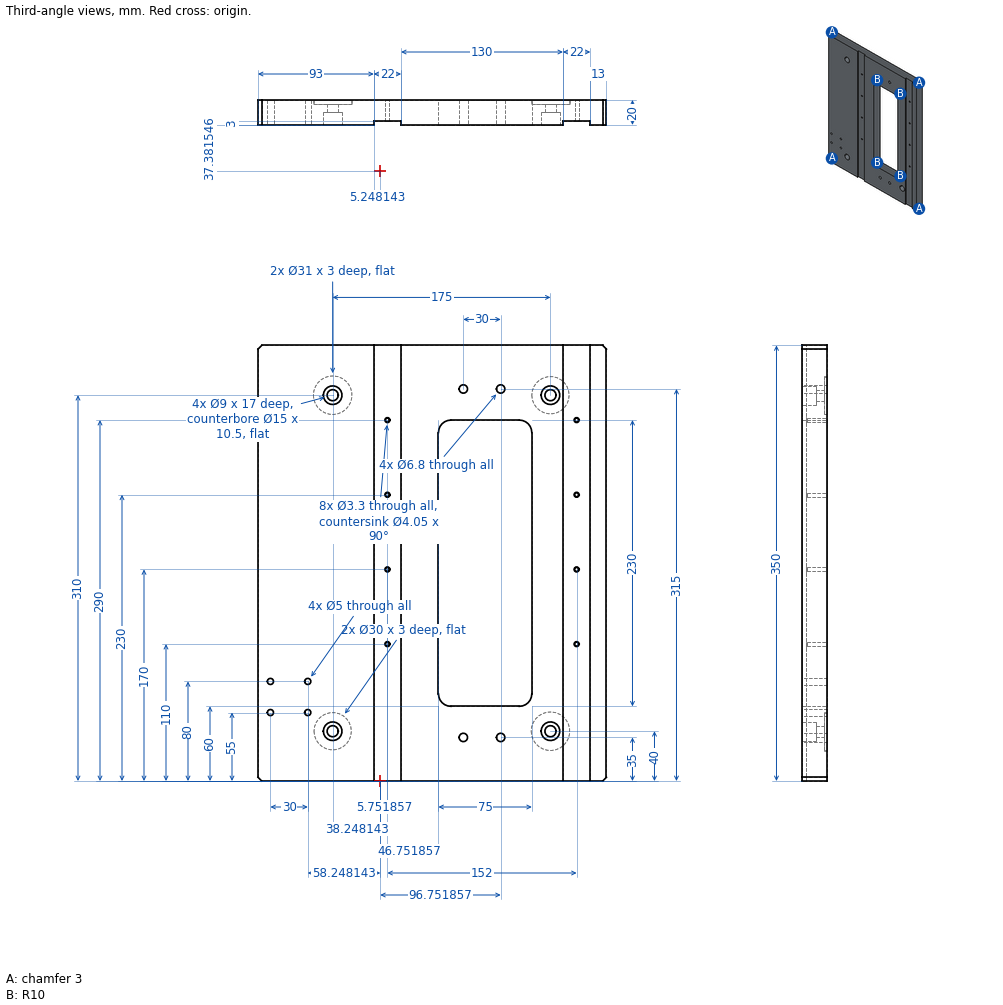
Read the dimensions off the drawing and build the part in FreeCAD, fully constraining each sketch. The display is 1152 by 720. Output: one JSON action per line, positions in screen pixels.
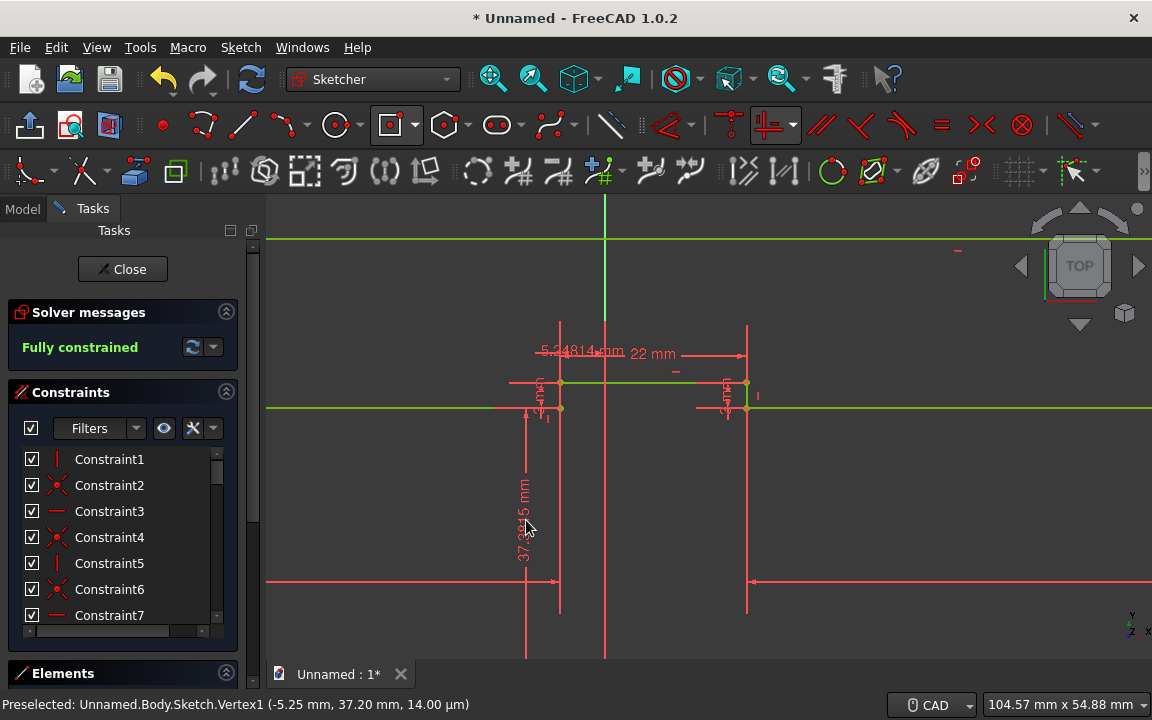
{"action": "left_click", "coordinate": [123, 269]}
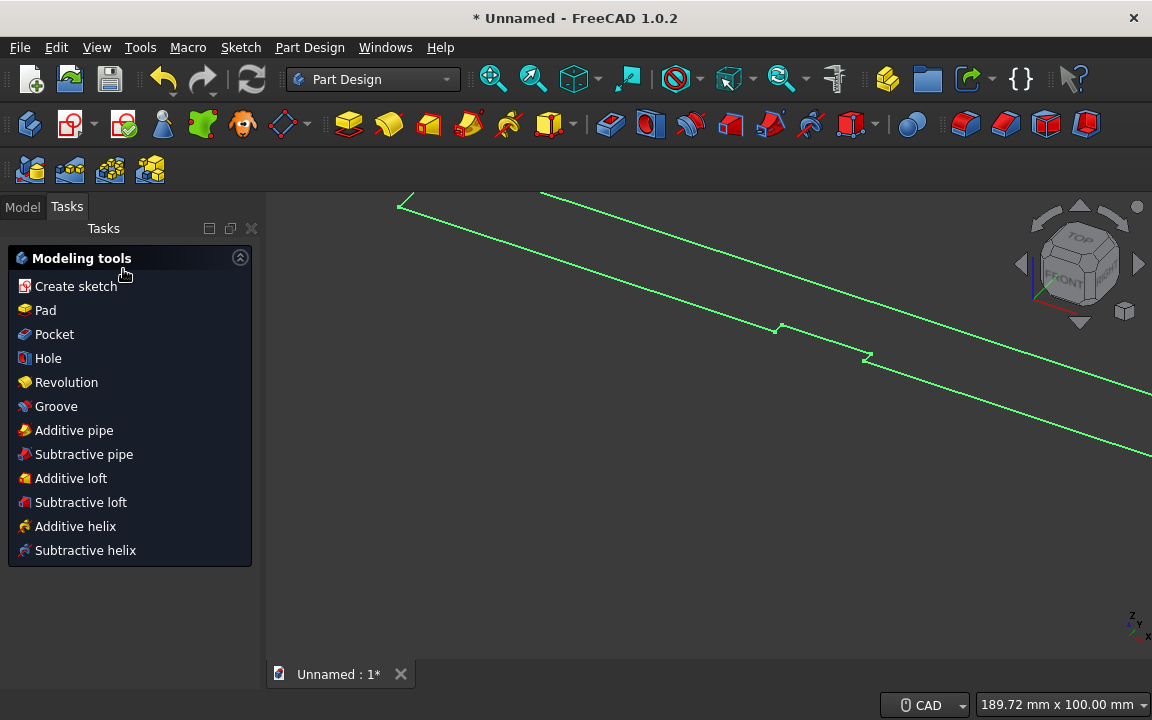
{"action": "left_click", "coordinate": [350, 124]}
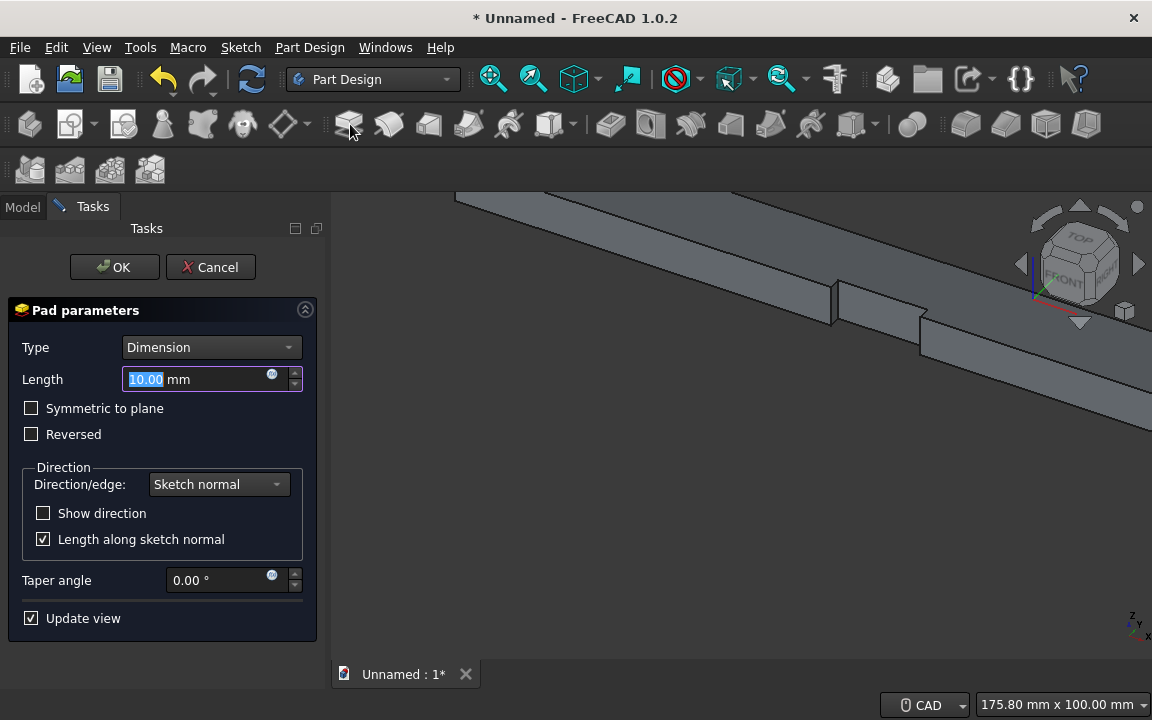
{"action": "type", "text": "350"}
{"action": "key", "text": "Tab"}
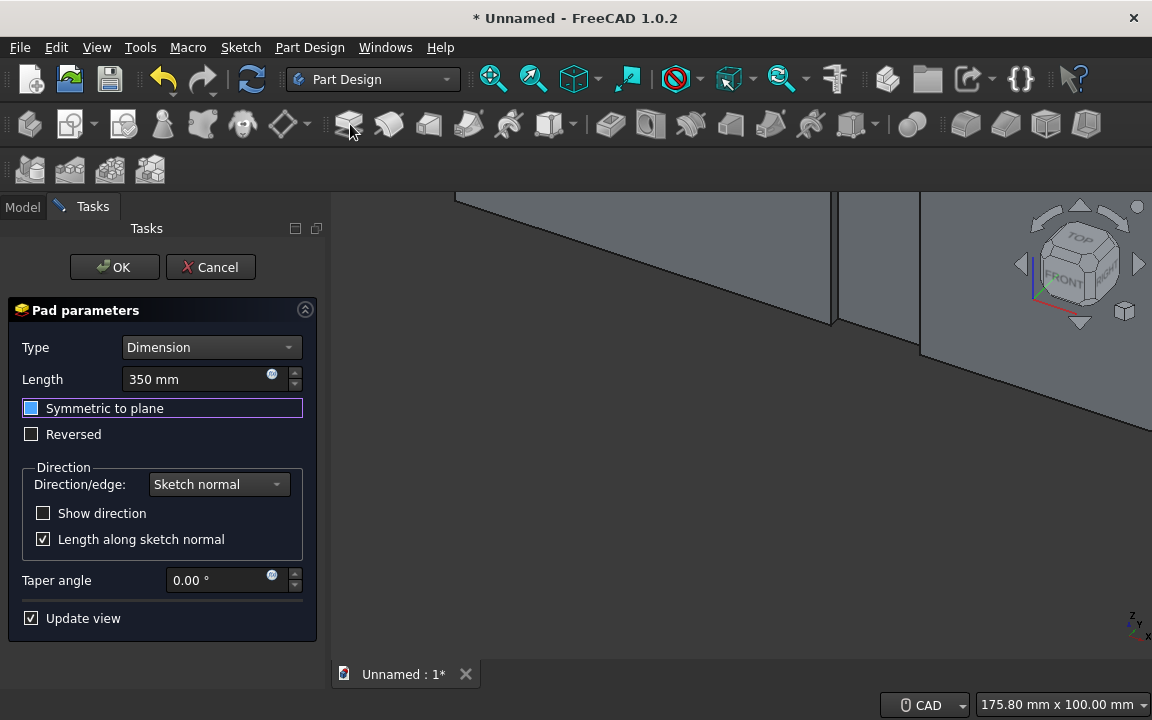
{"action": "left_click", "coordinate": [115, 267]}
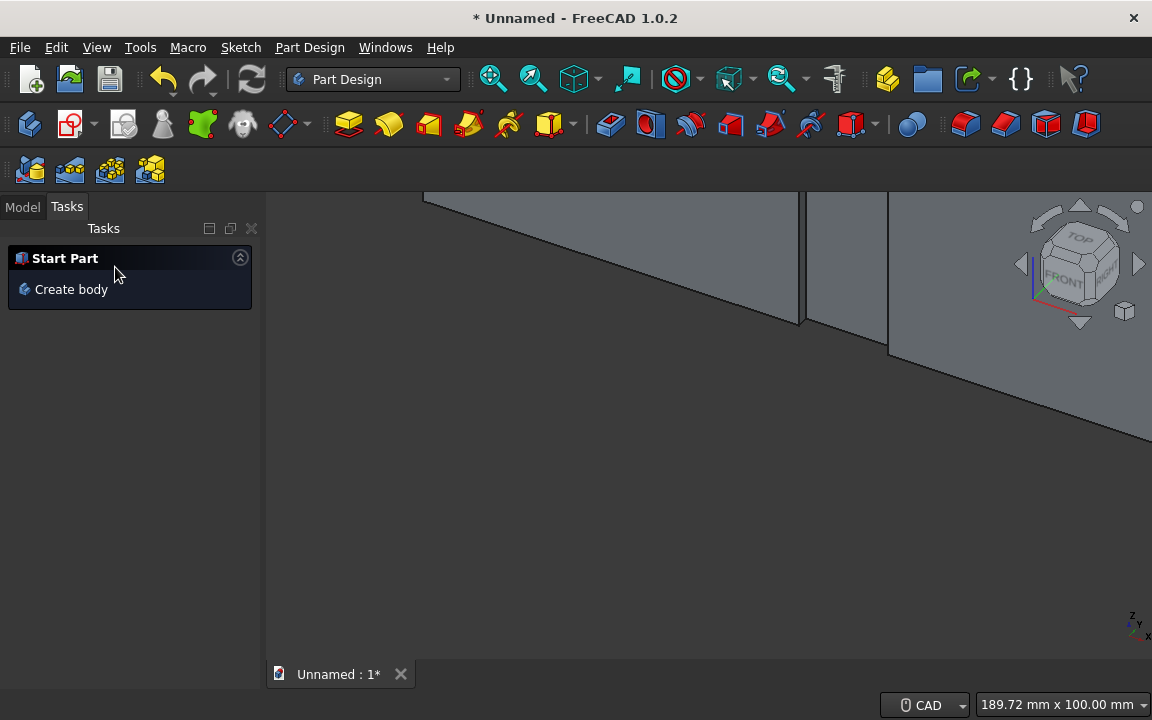
{"action": "left_click", "coordinate": [494, 80]}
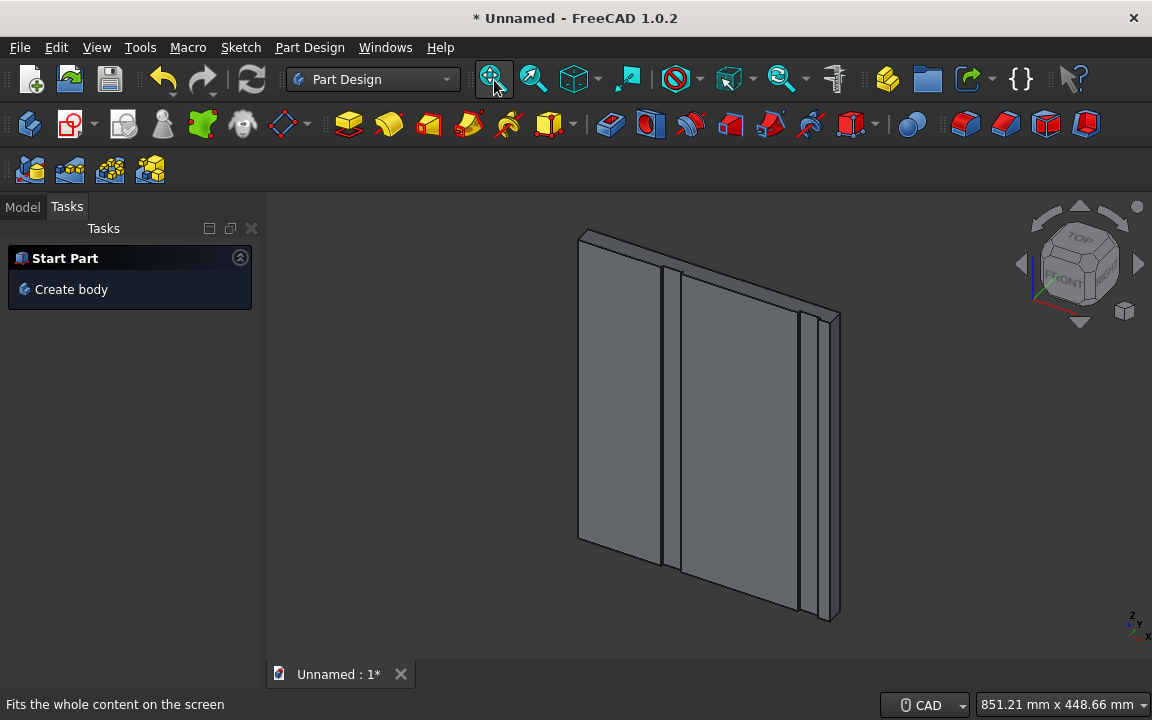
{"action": "left_click", "coordinate": [835, 317]}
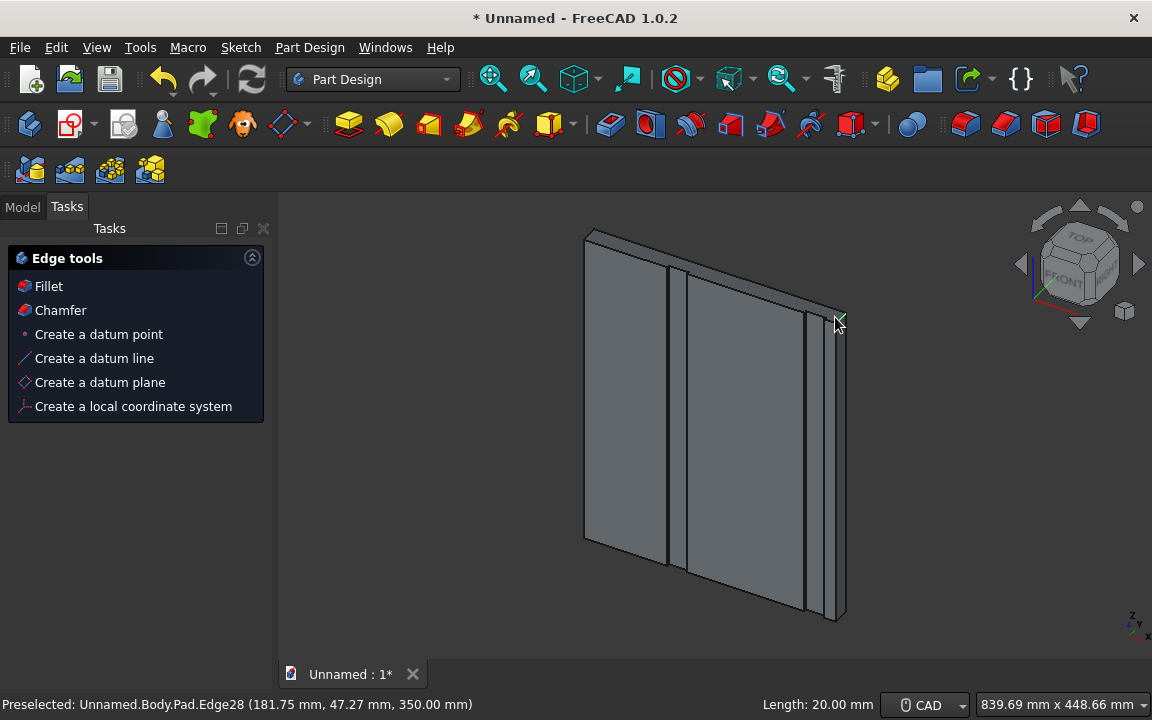
{"action": "scroll", "coordinate": [841, 616], "scroll_direction": "up", "scroll_amount": 4}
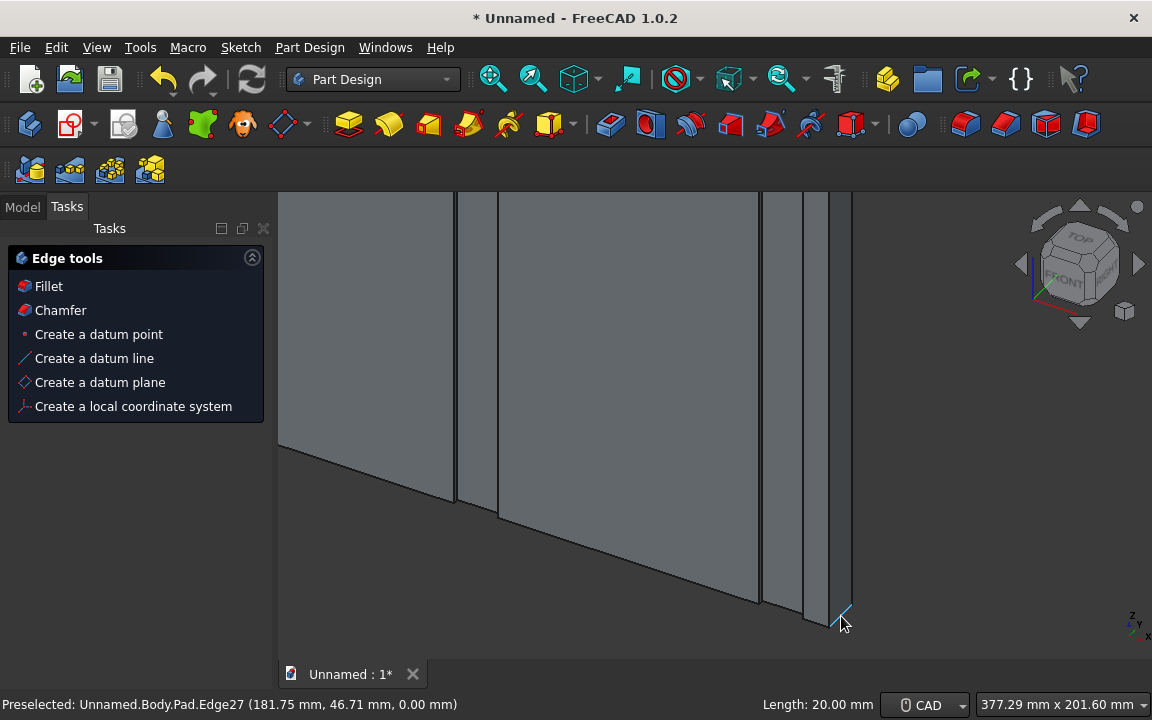
{"action": "left_click", "coordinate": [494, 80]}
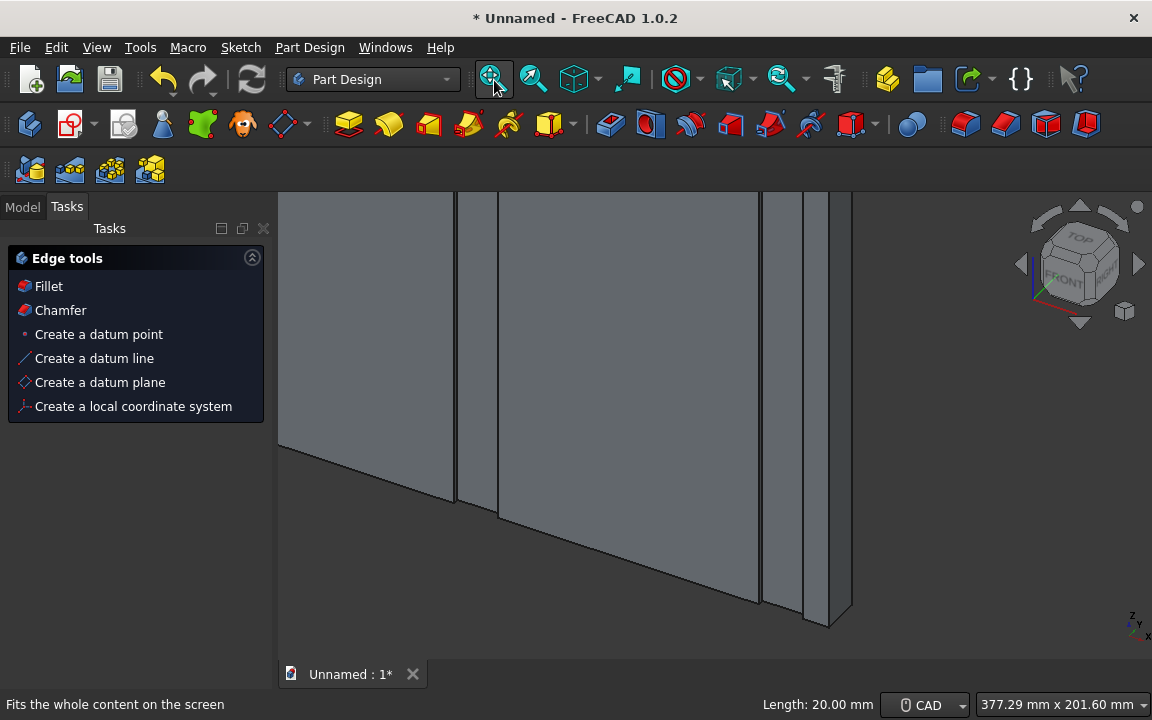
{"action": "key", "text": "0"}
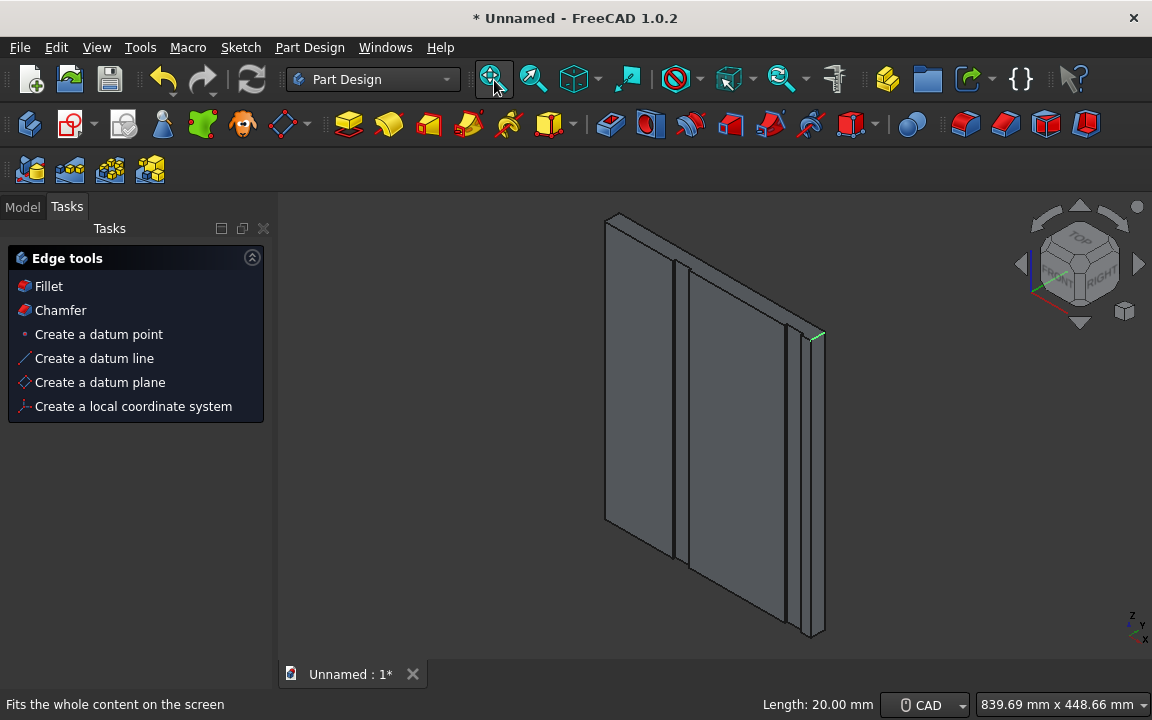
{"action": "key", "text": "2"}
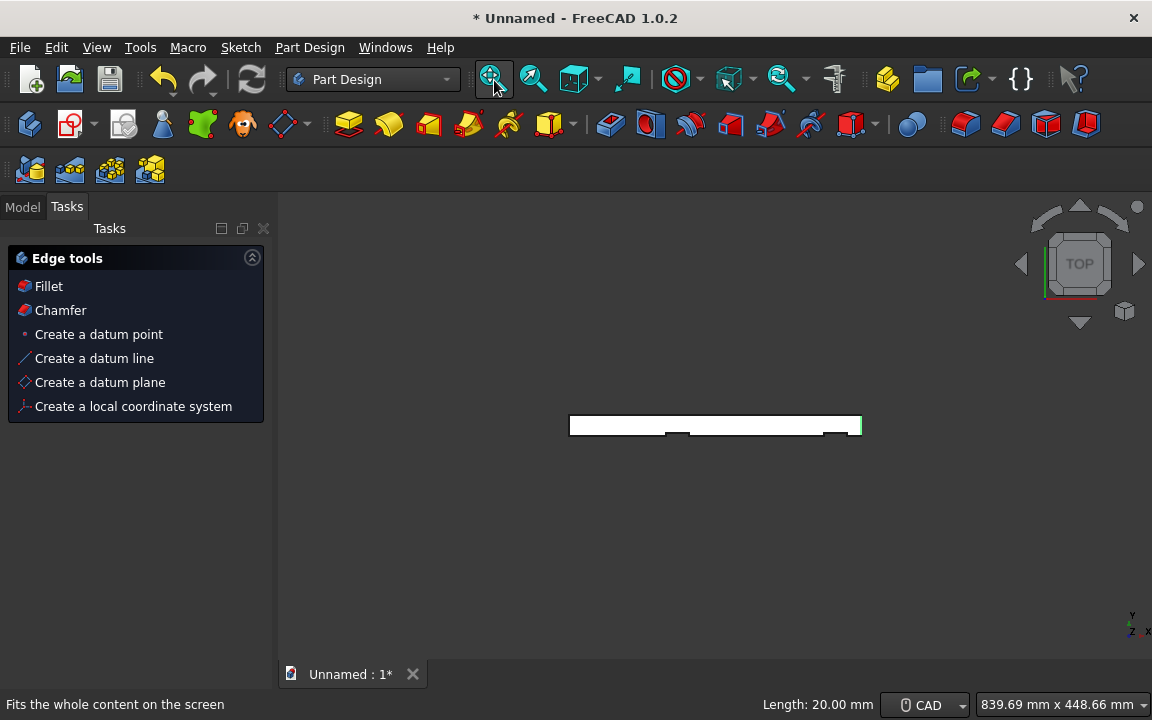
{"action": "left_click", "coordinate": [494, 80]}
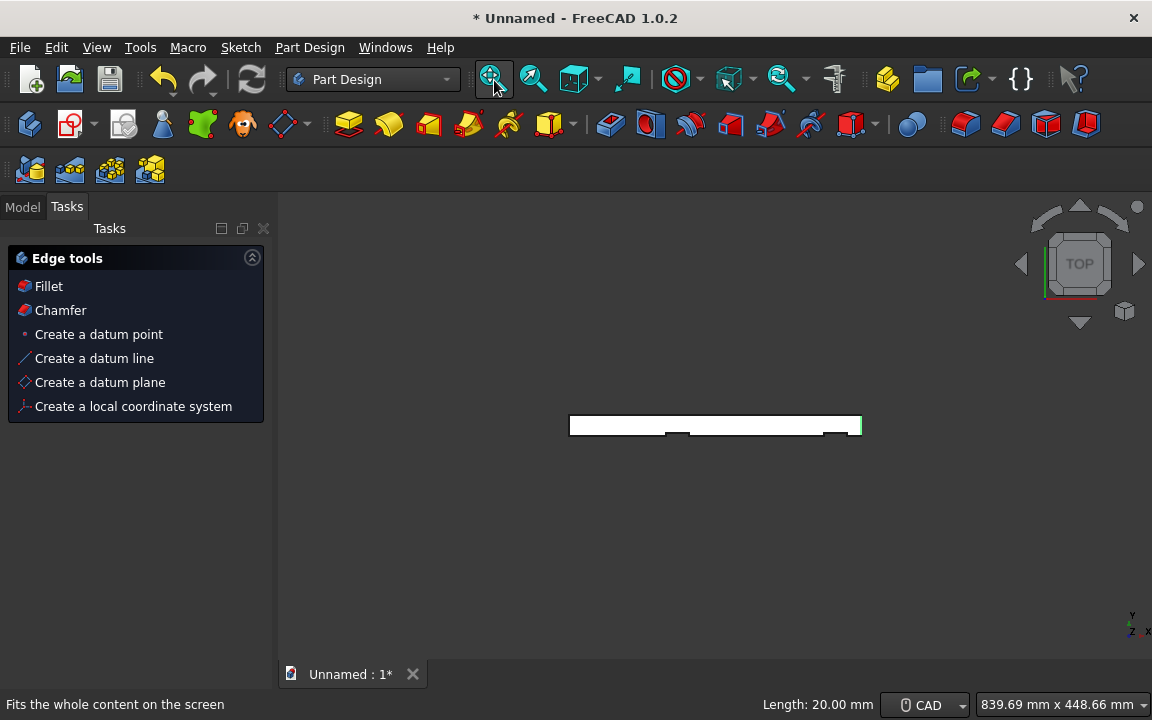
{"action": "left_click", "coordinate": [569, 424], "text": "ctrl"}